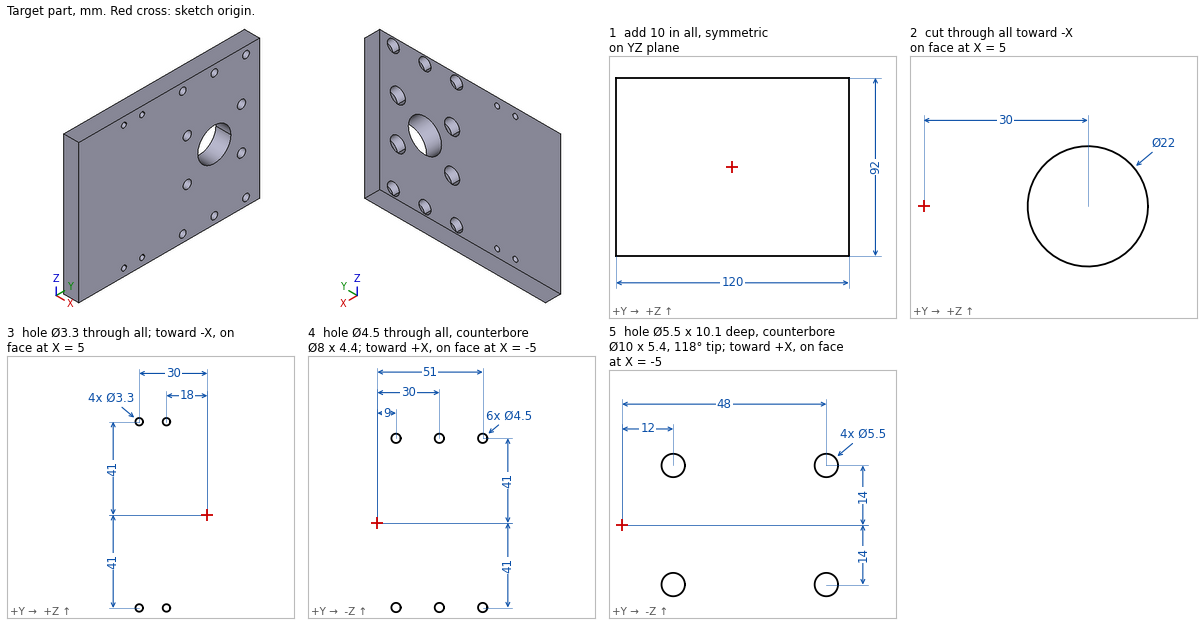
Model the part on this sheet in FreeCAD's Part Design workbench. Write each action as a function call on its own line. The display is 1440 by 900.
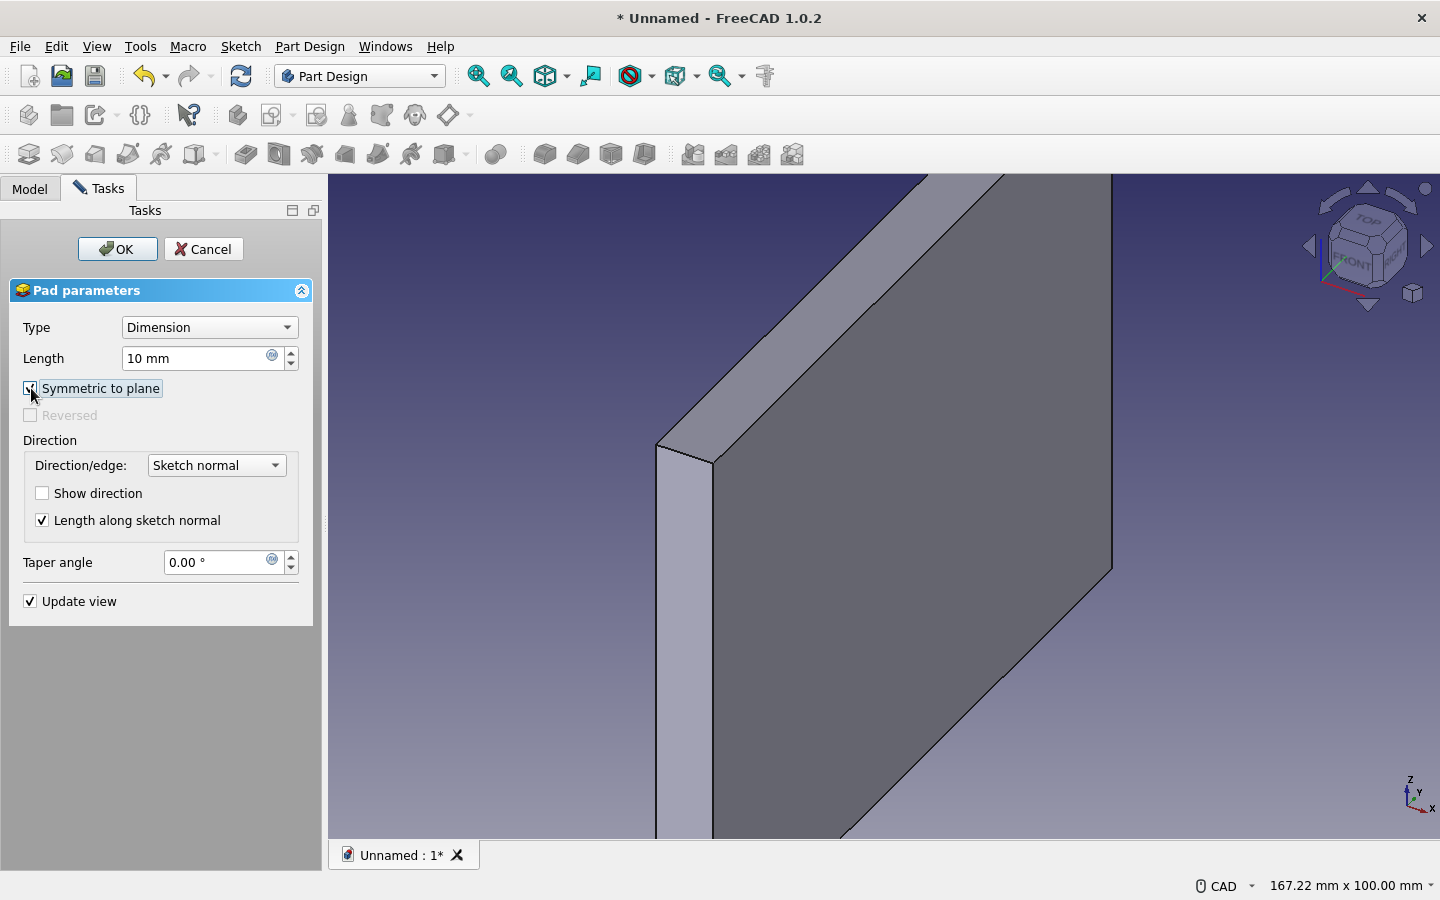
click(118, 249)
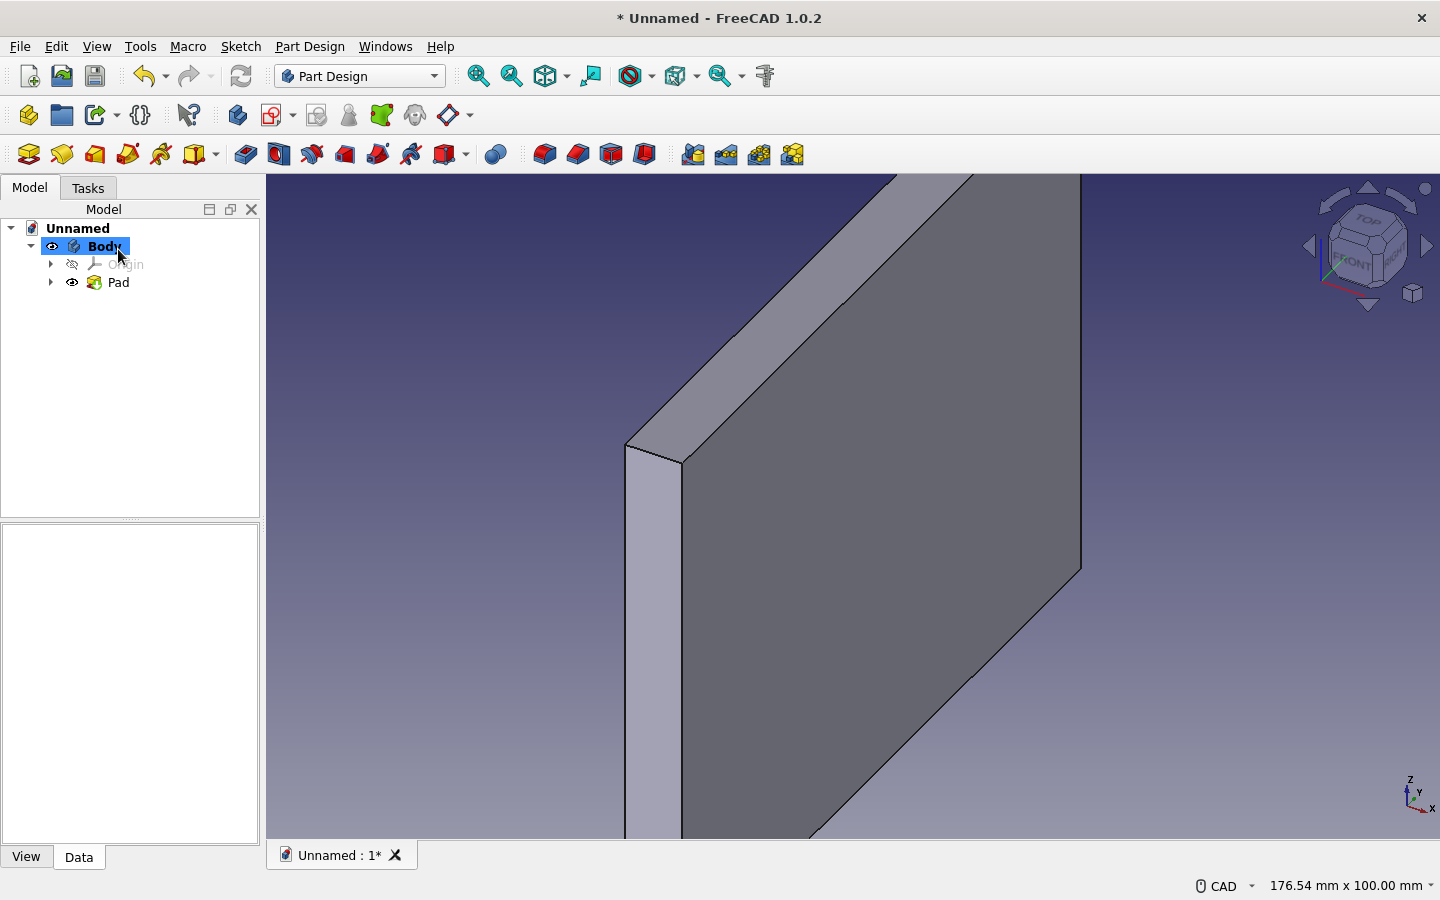
click(479, 76)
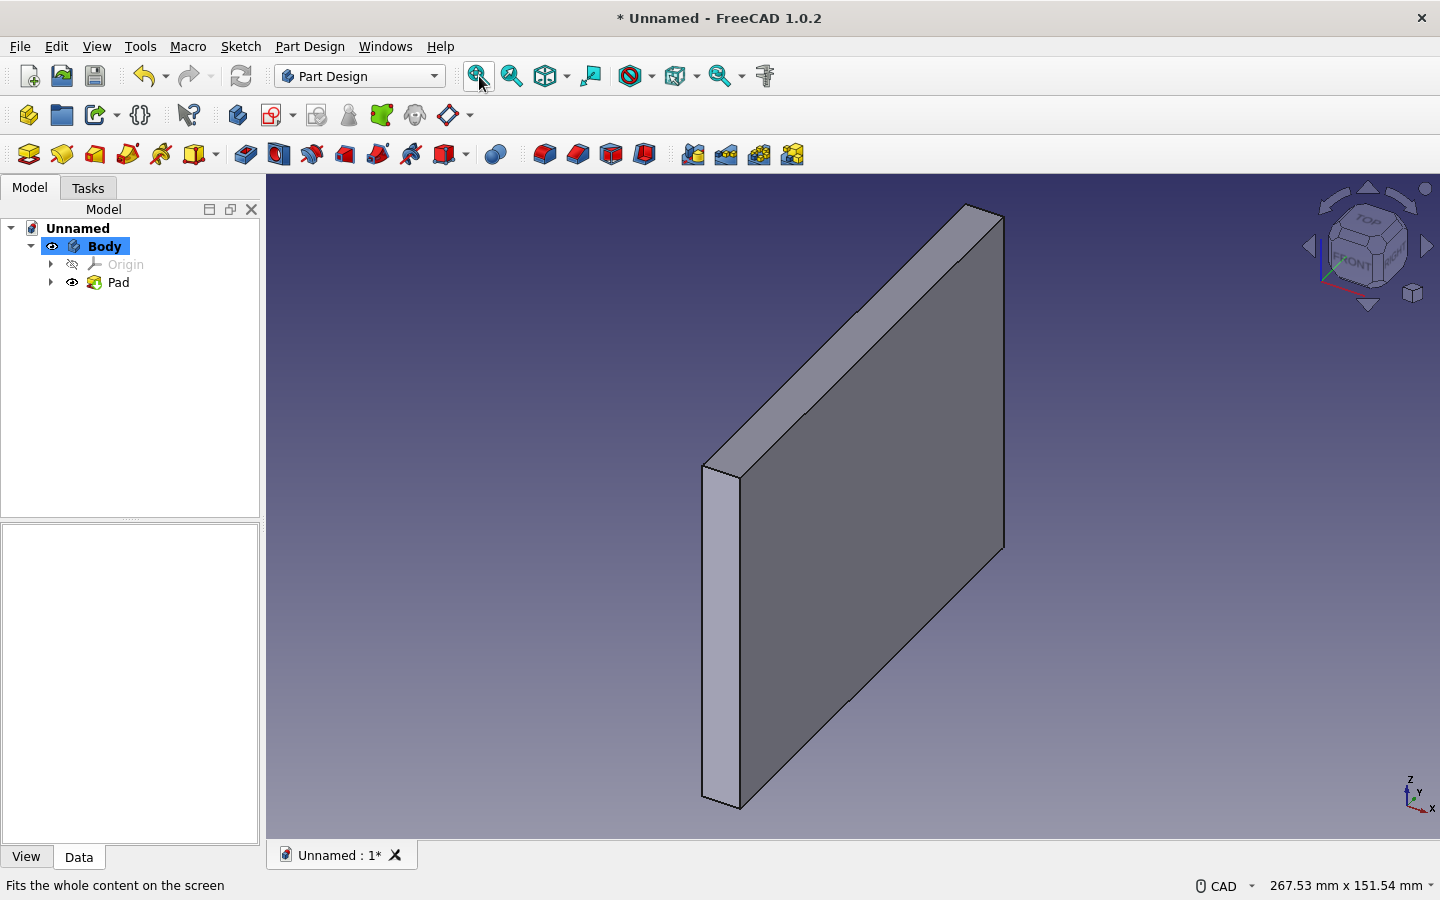
click(872, 512)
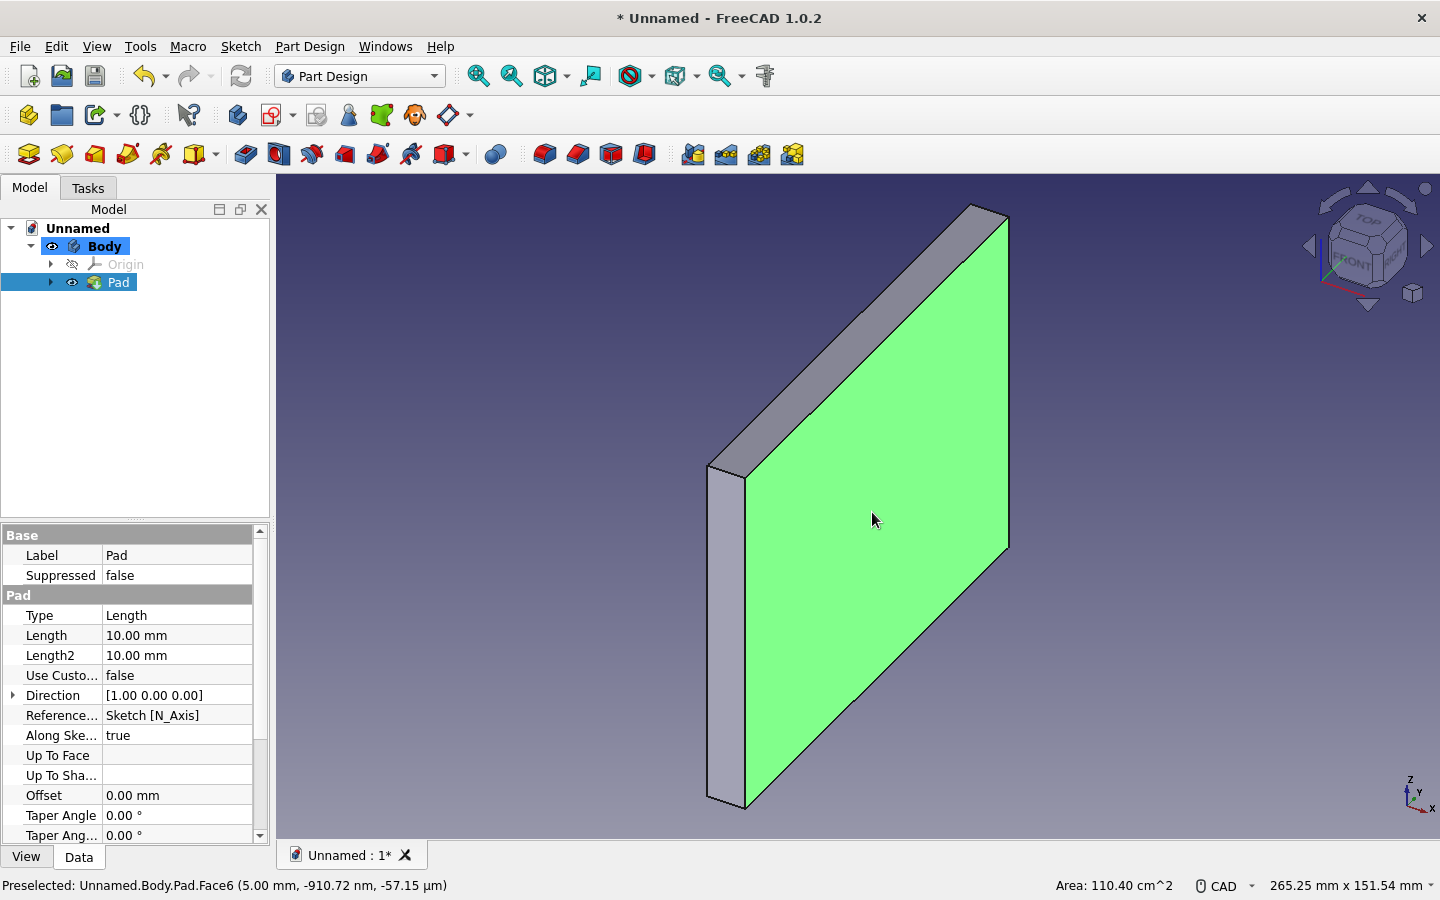
click(270, 116)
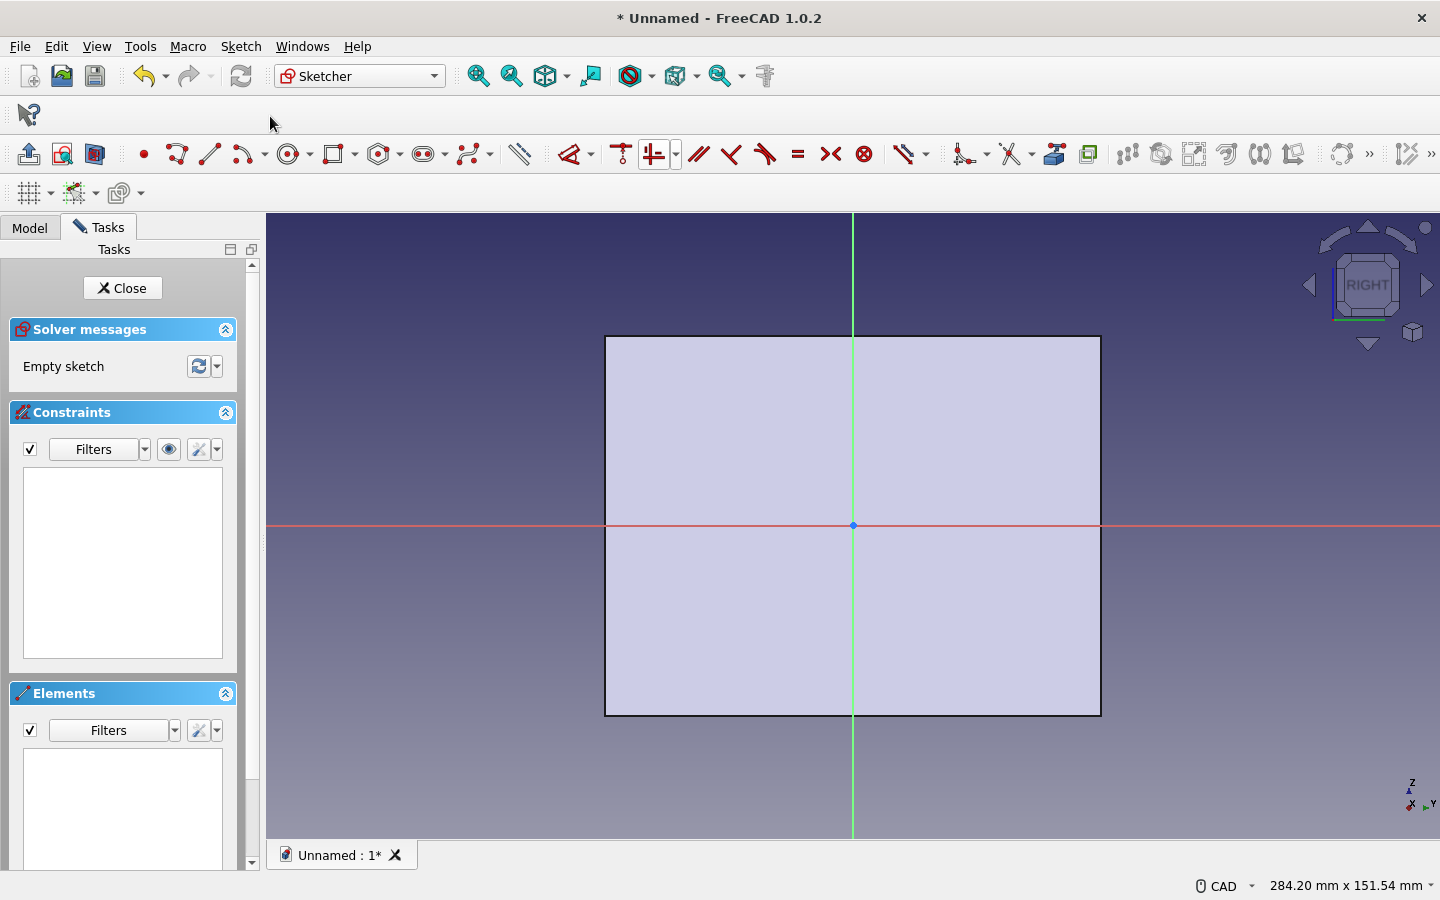
scroll(988, 526, up, 7)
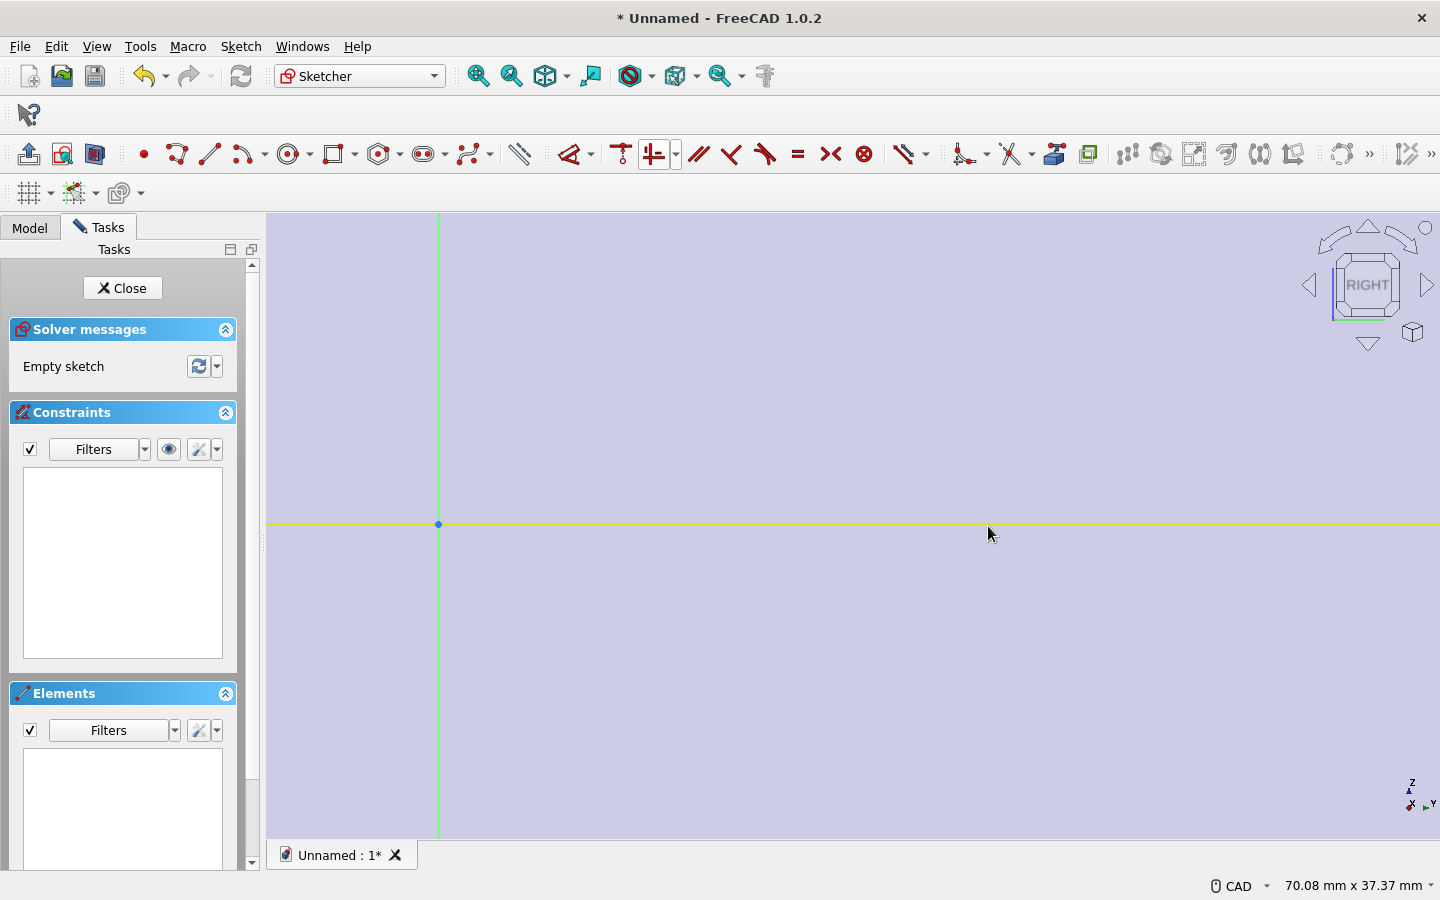
key(g)
key(c)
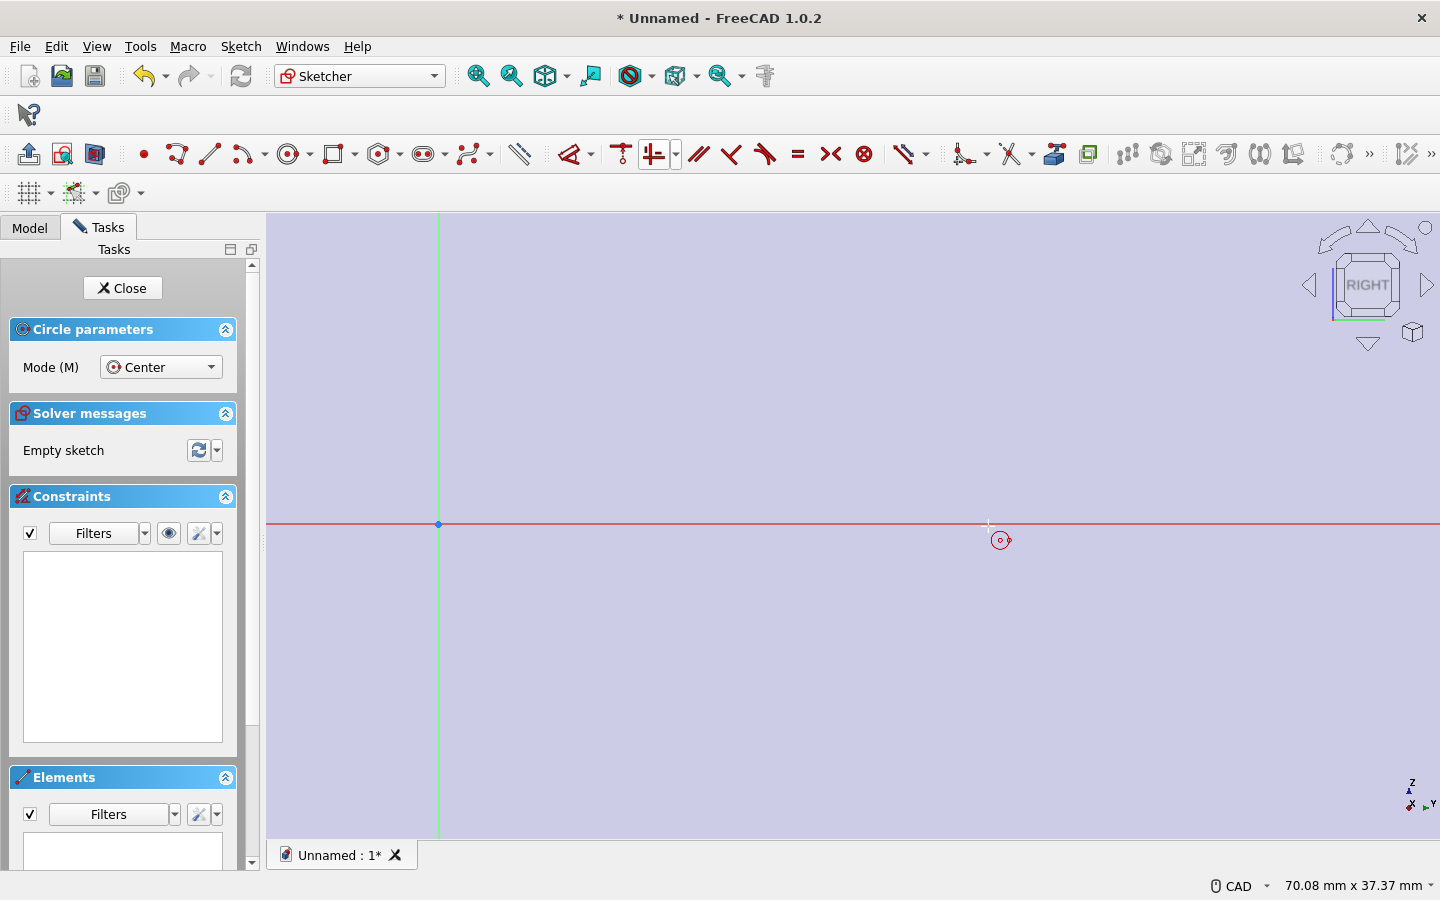
click(941, 524)
click(1072, 394)
key(Escape)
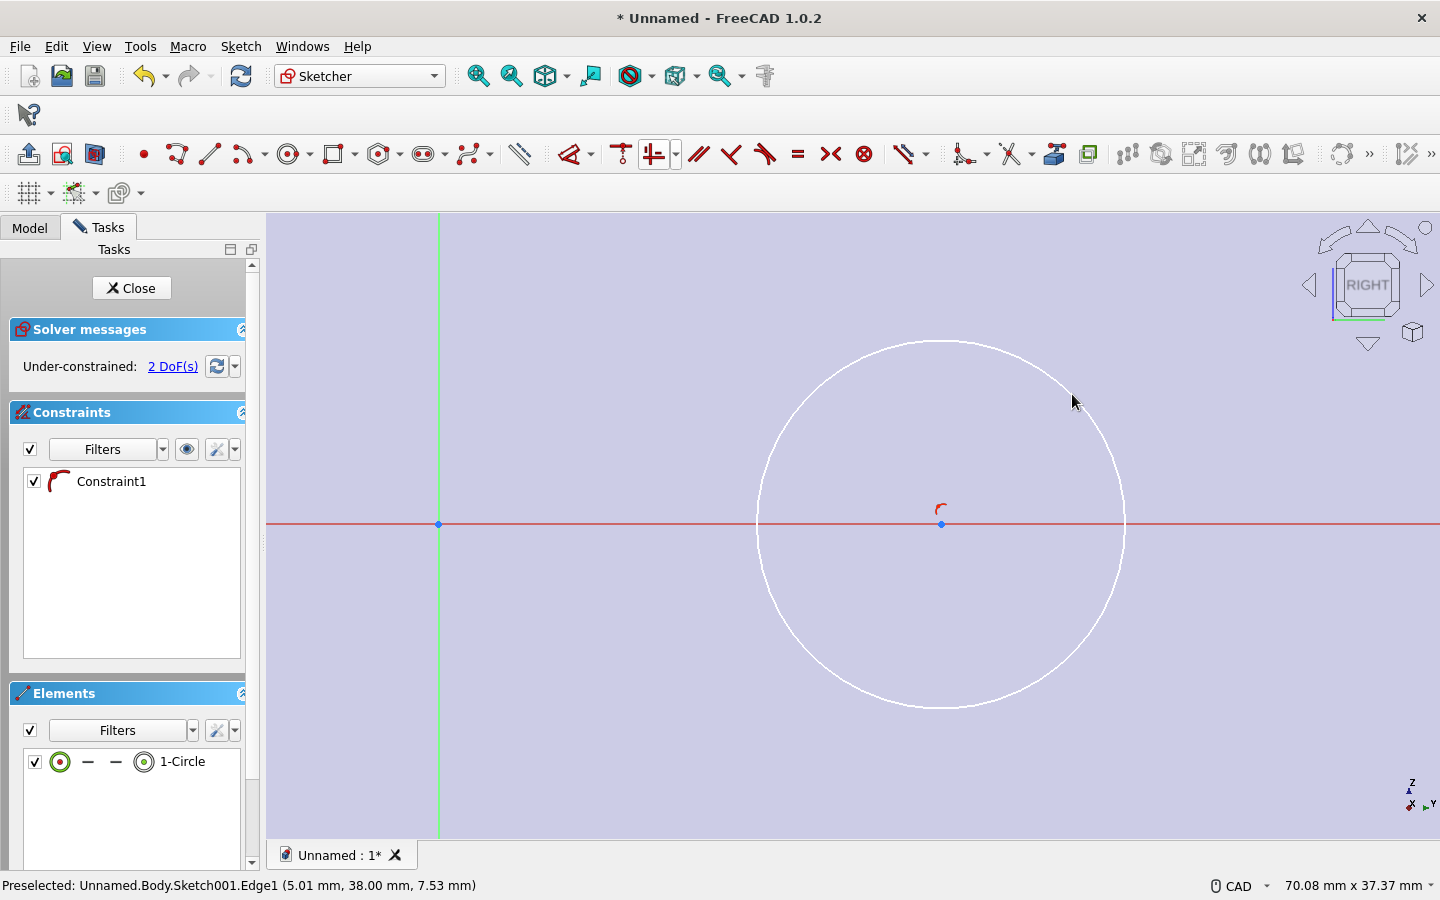
key(d)